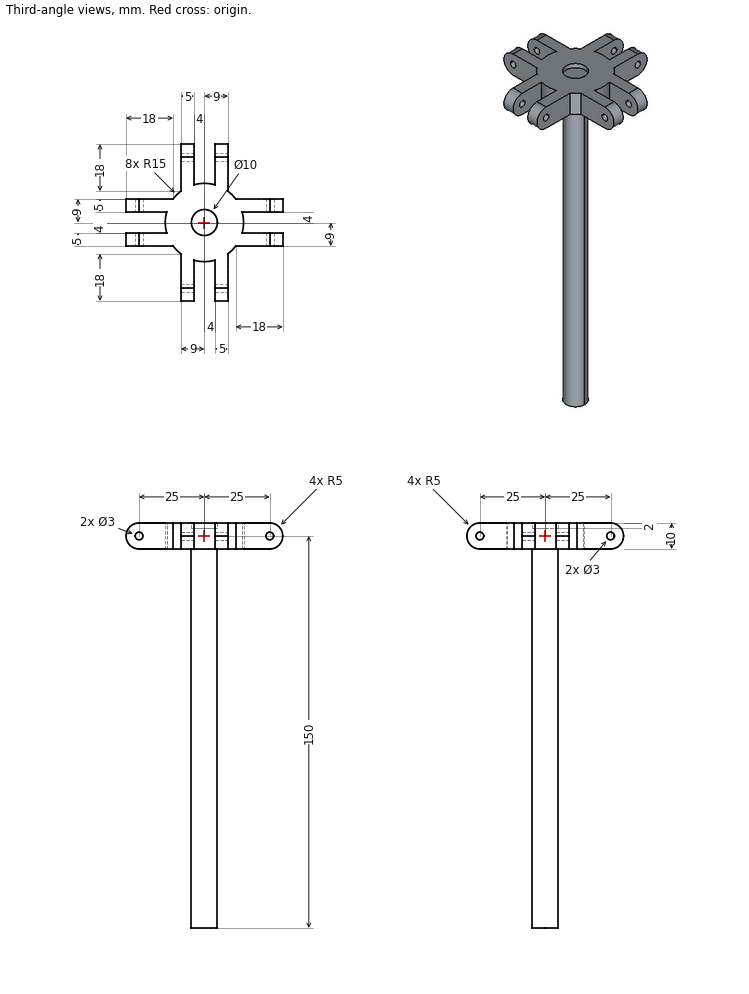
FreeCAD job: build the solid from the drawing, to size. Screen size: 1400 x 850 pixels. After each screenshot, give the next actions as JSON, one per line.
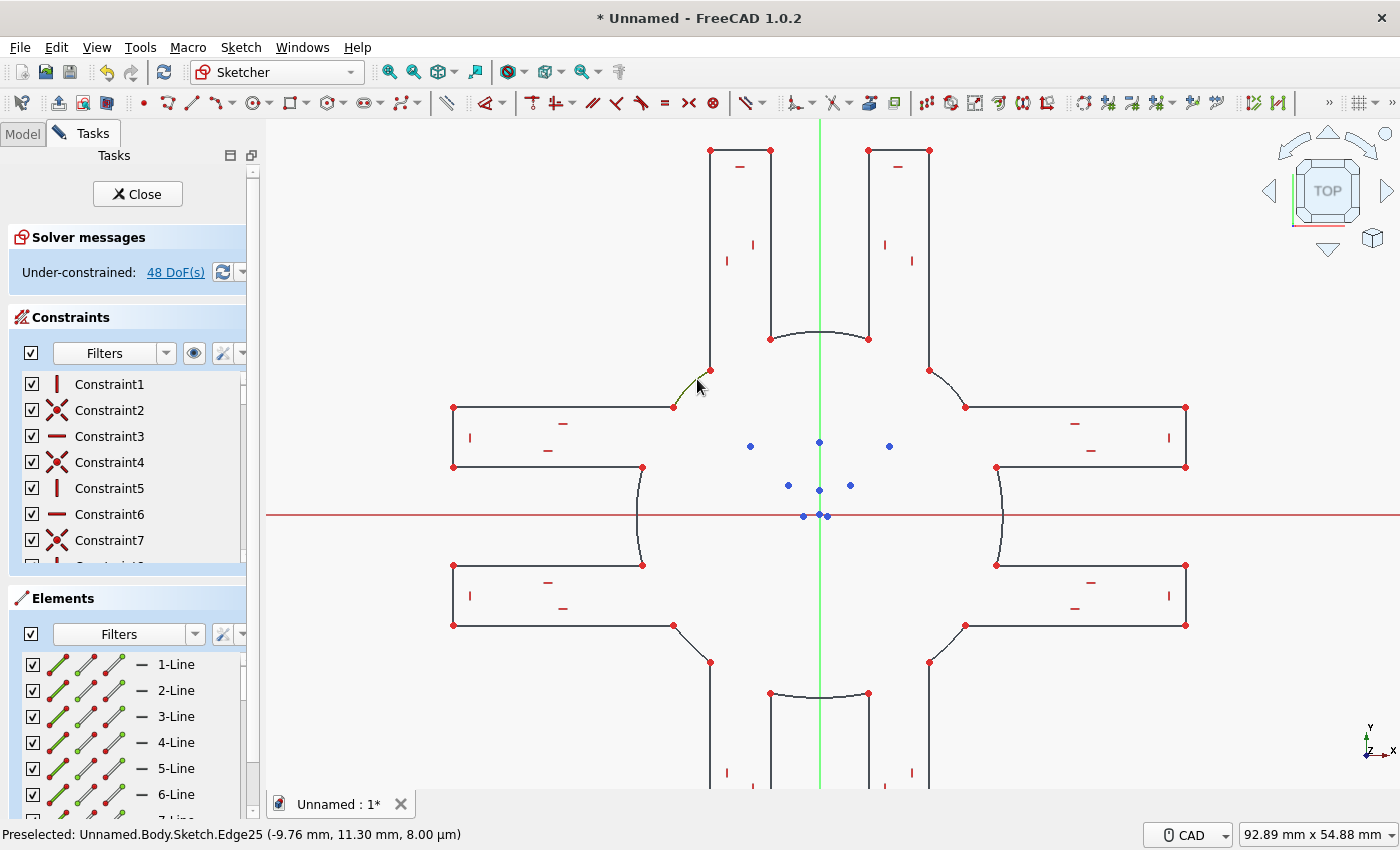
{"action": "left_click", "coordinate": [638, 496]}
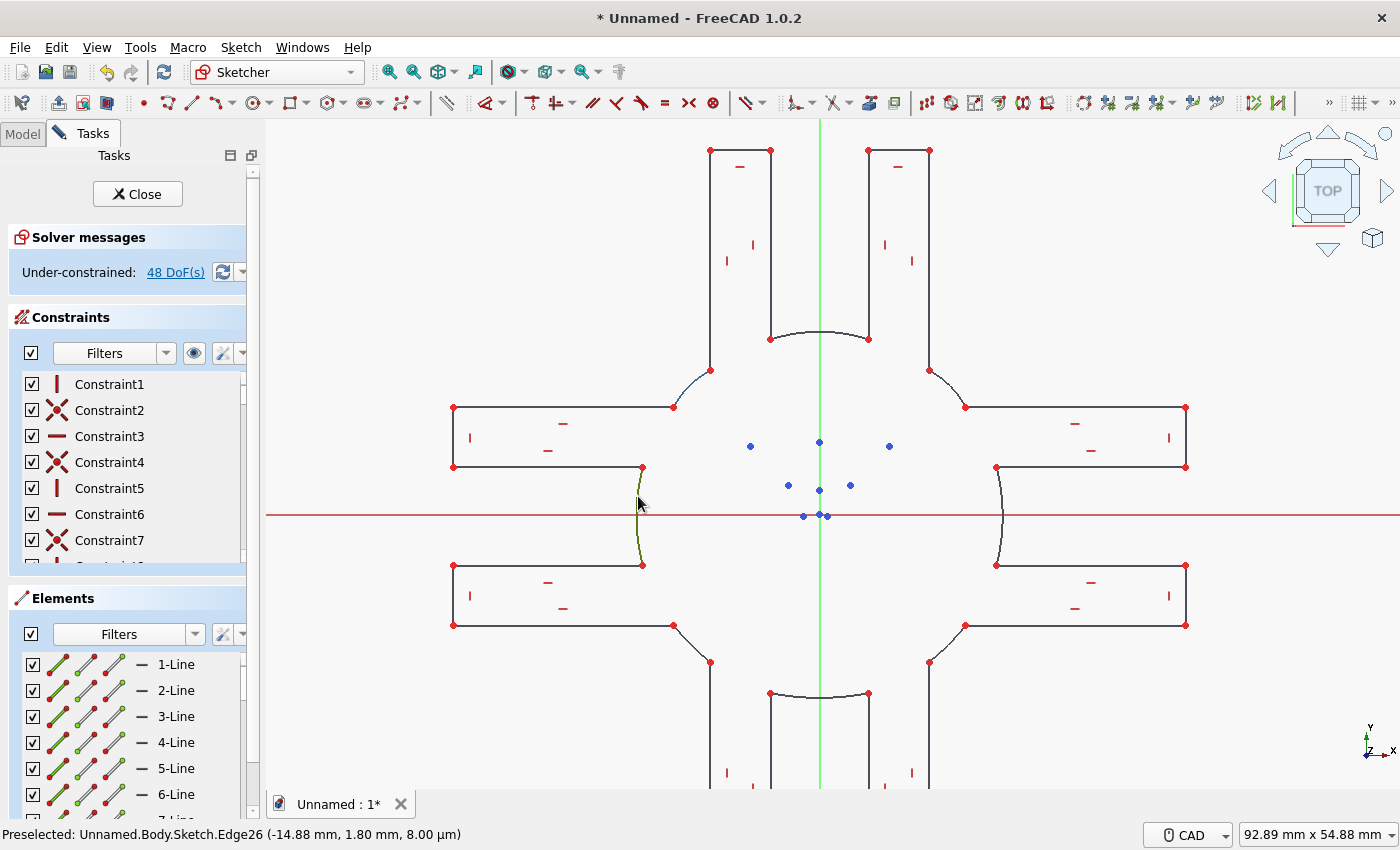
{"action": "left_click", "coordinate": [532, 104]}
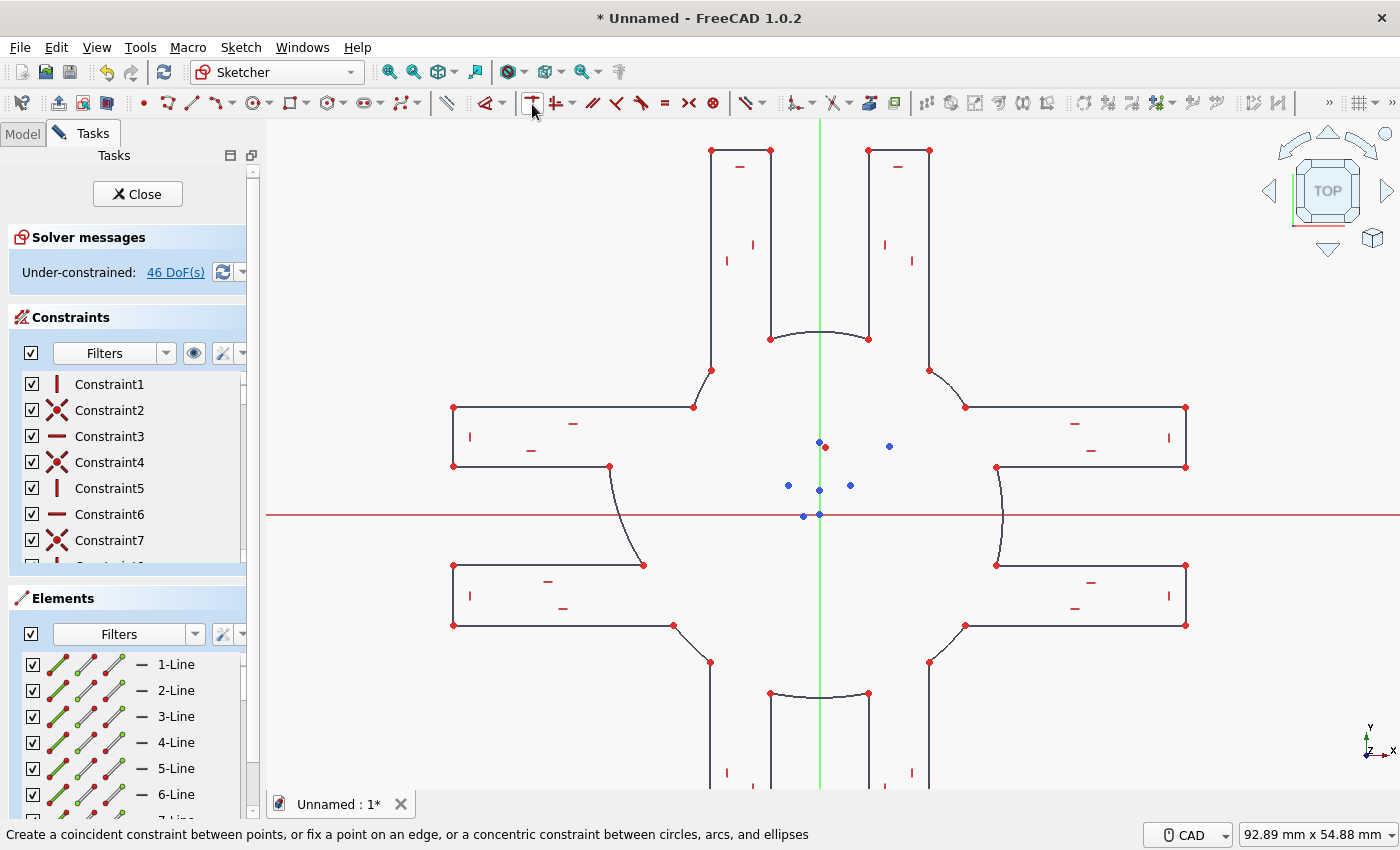
{"action": "left_click", "coordinate": [705, 381]}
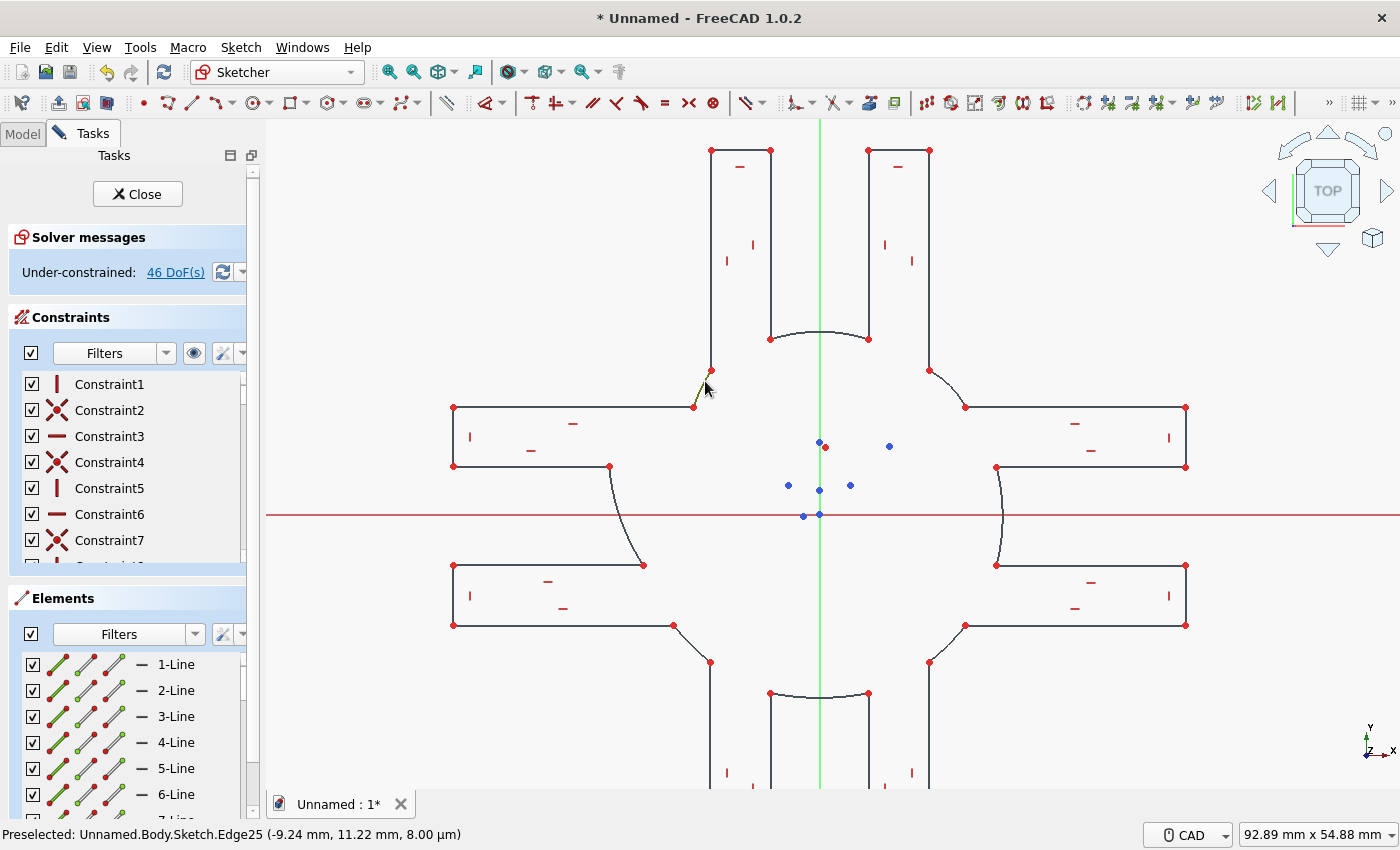
{"action": "left_click", "coordinate": [684, 637]}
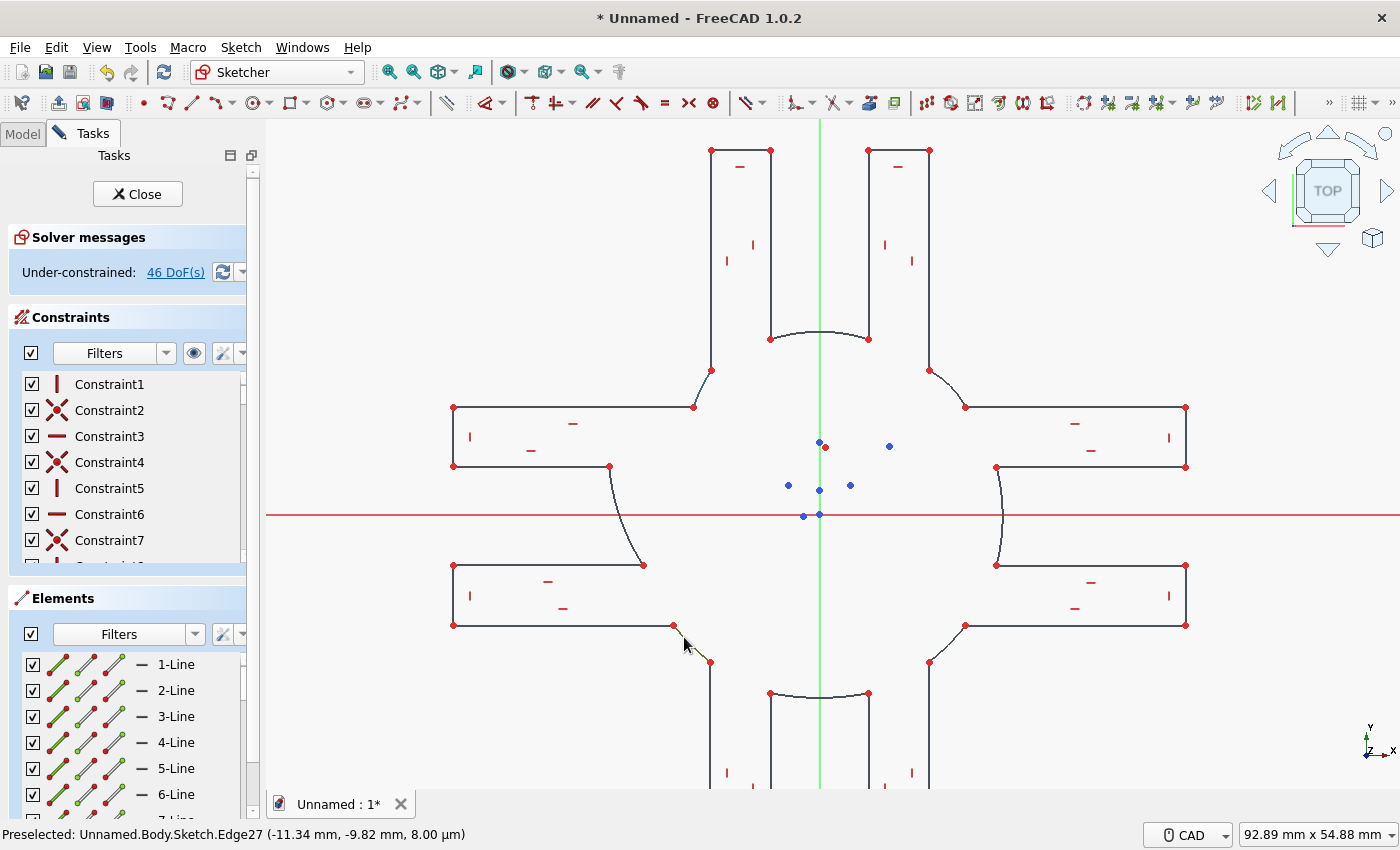
{"action": "key", "text": "c"}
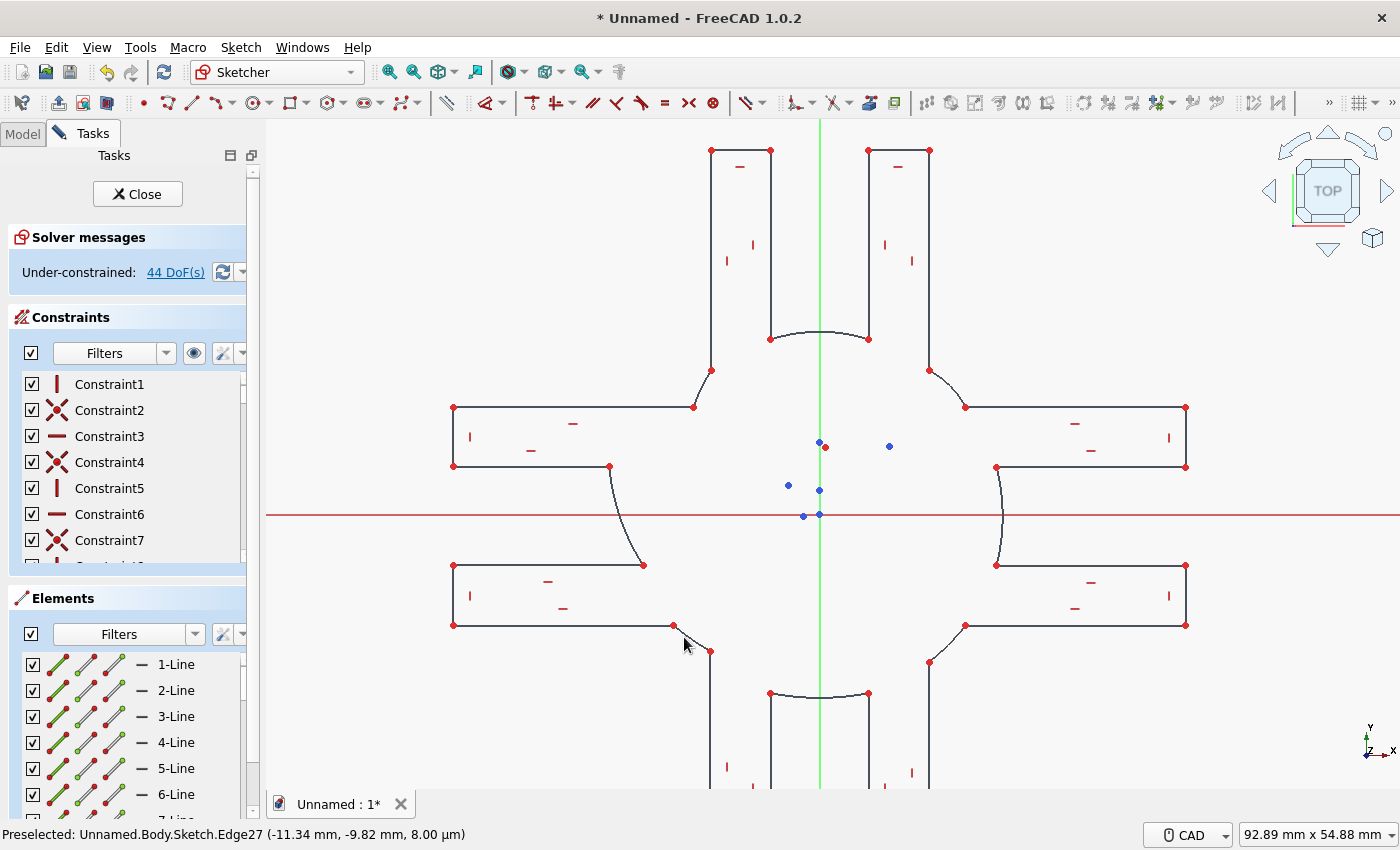
{"action": "left_click", "coordinate": [705, 381]}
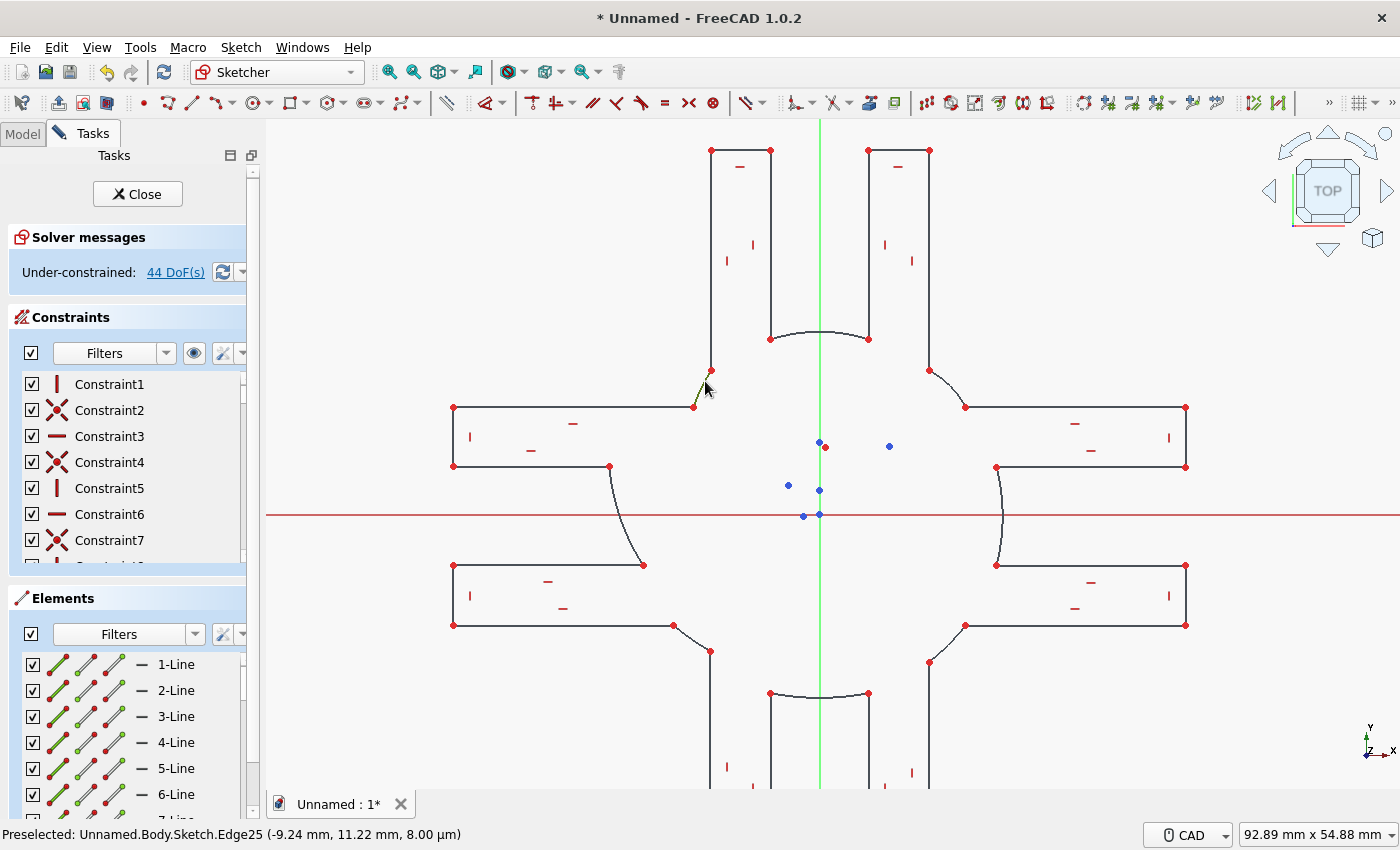
{"action": "left_click", "coordinate": [800, 697]}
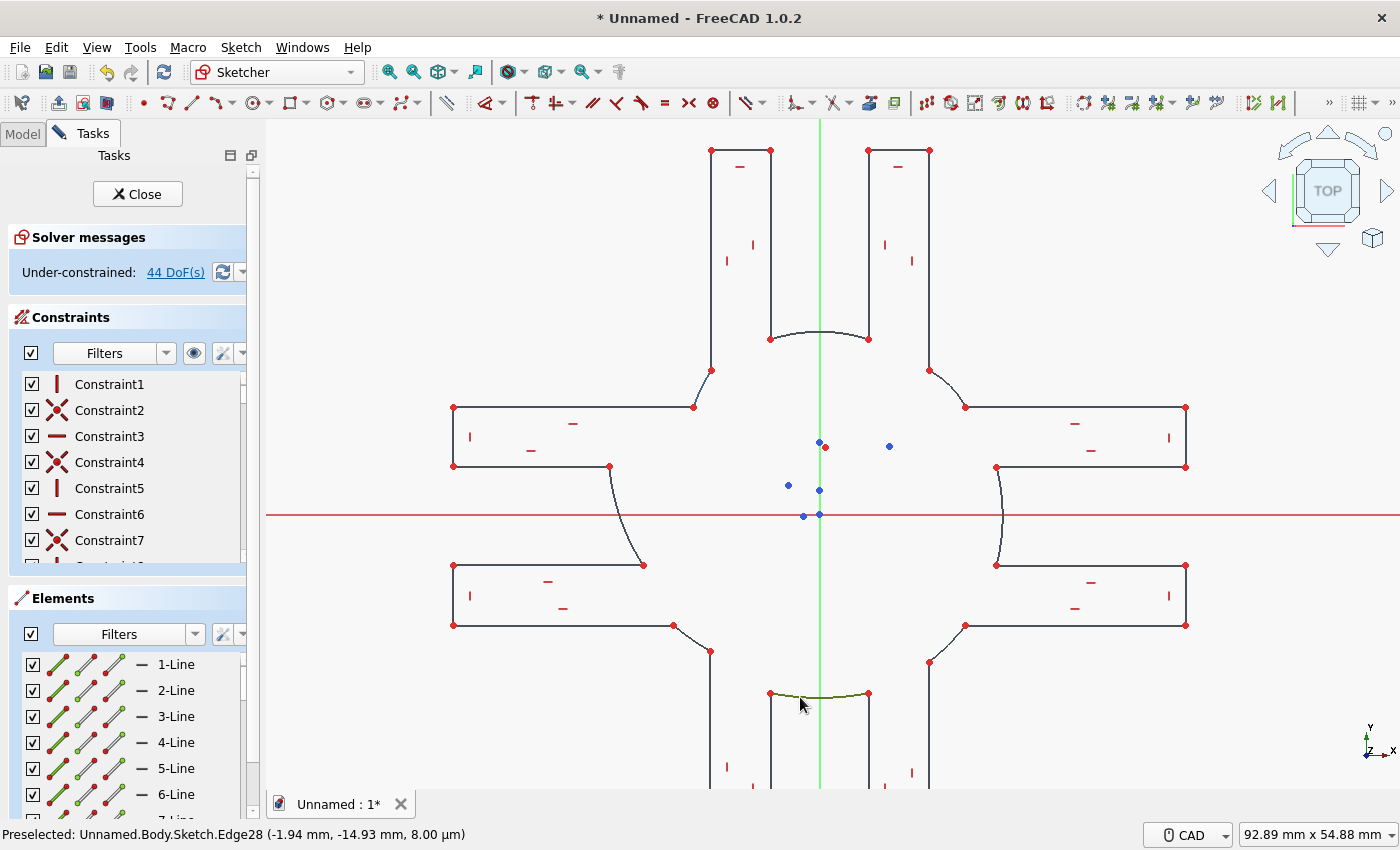
{"action": "key", "text": "c"}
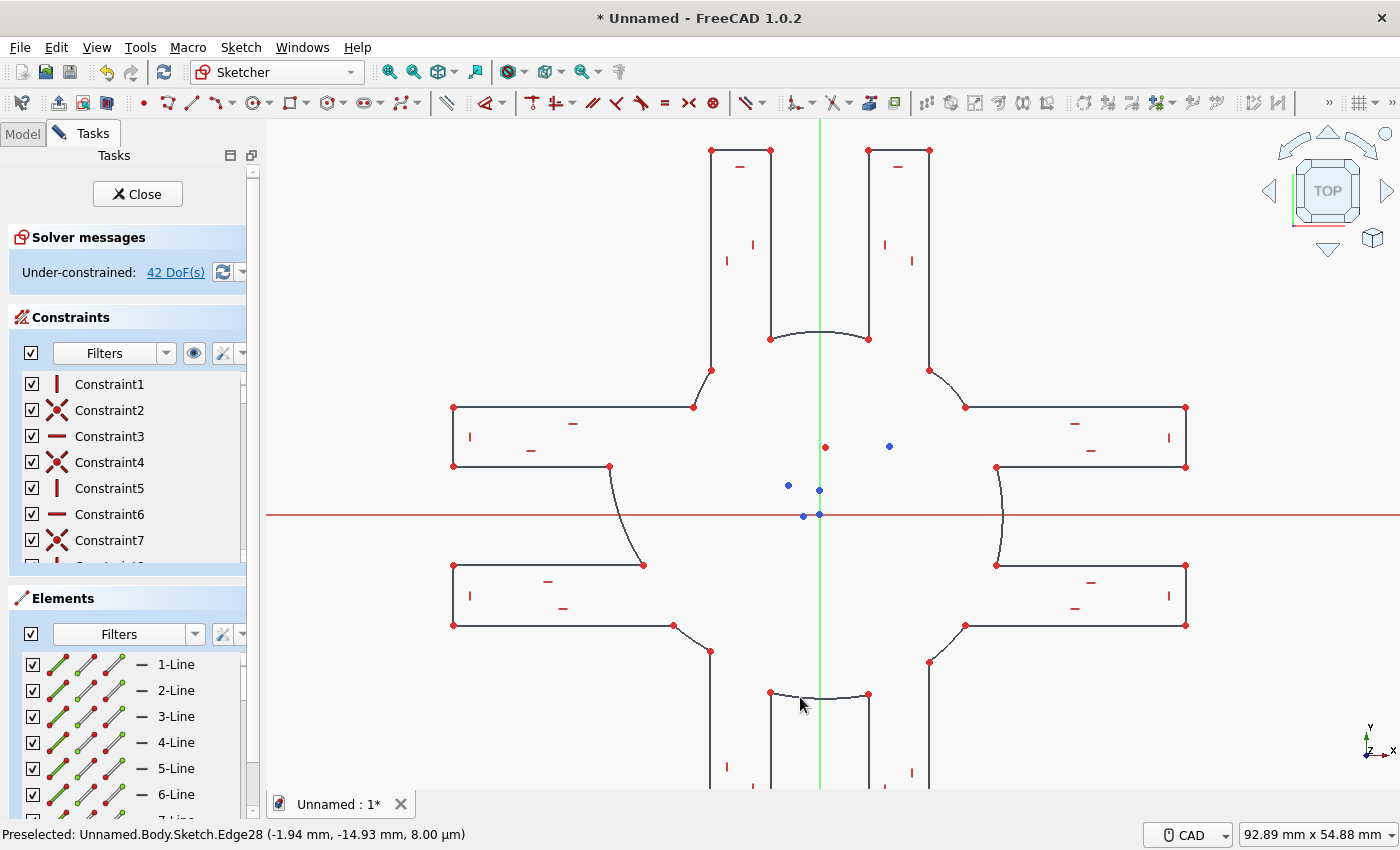
{"action": "left_click", "coordinate": [705, 381]}